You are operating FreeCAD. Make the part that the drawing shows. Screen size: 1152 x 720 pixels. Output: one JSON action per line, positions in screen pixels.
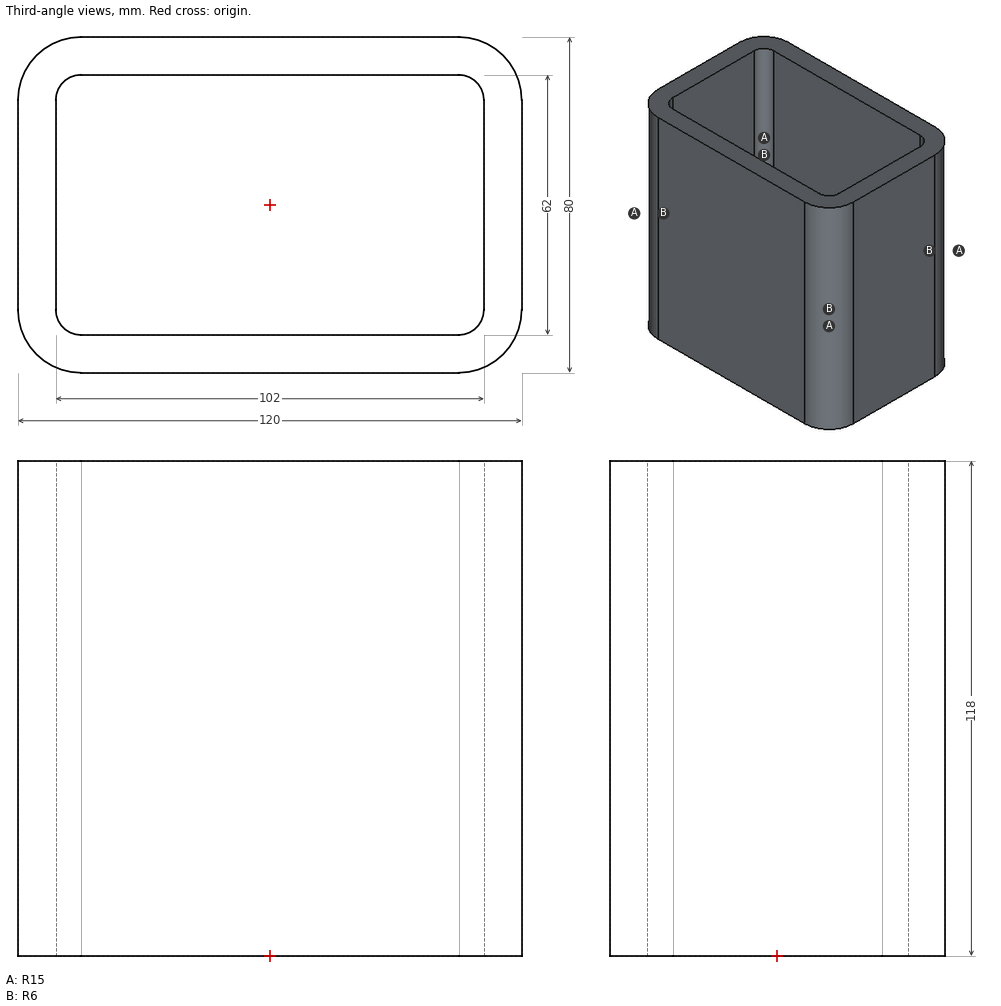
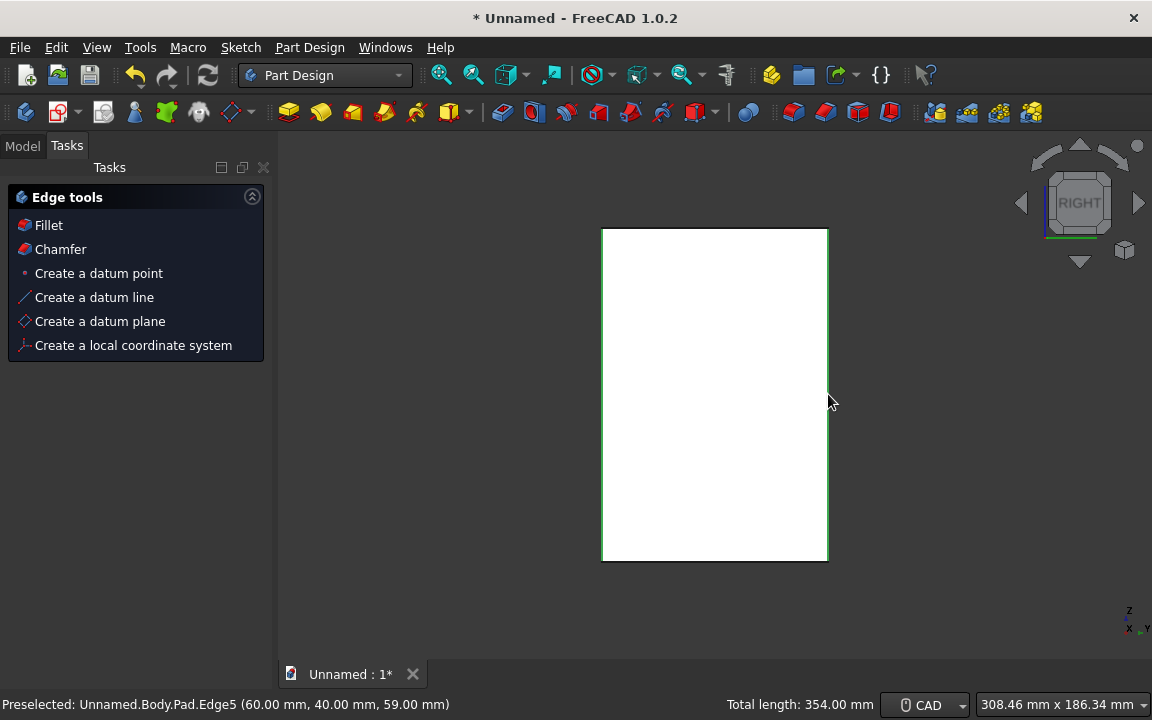
{"action": "key", "text": "5"}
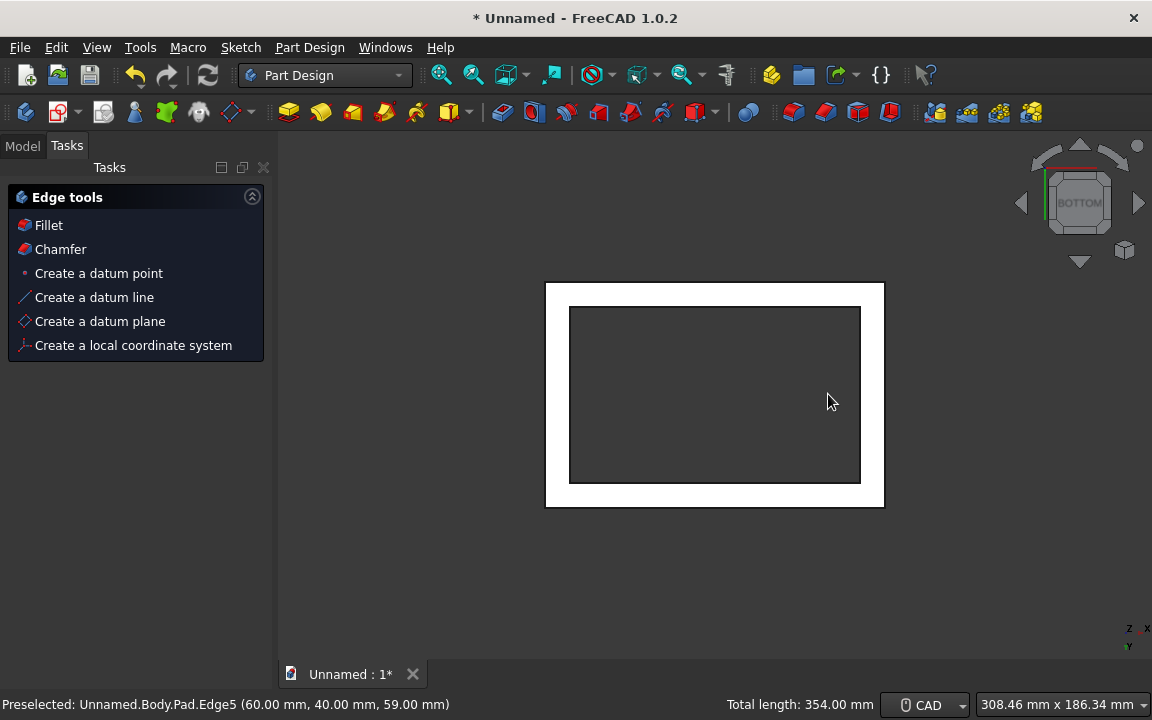
{"action": "left_click", "coordinate": [442, 76]}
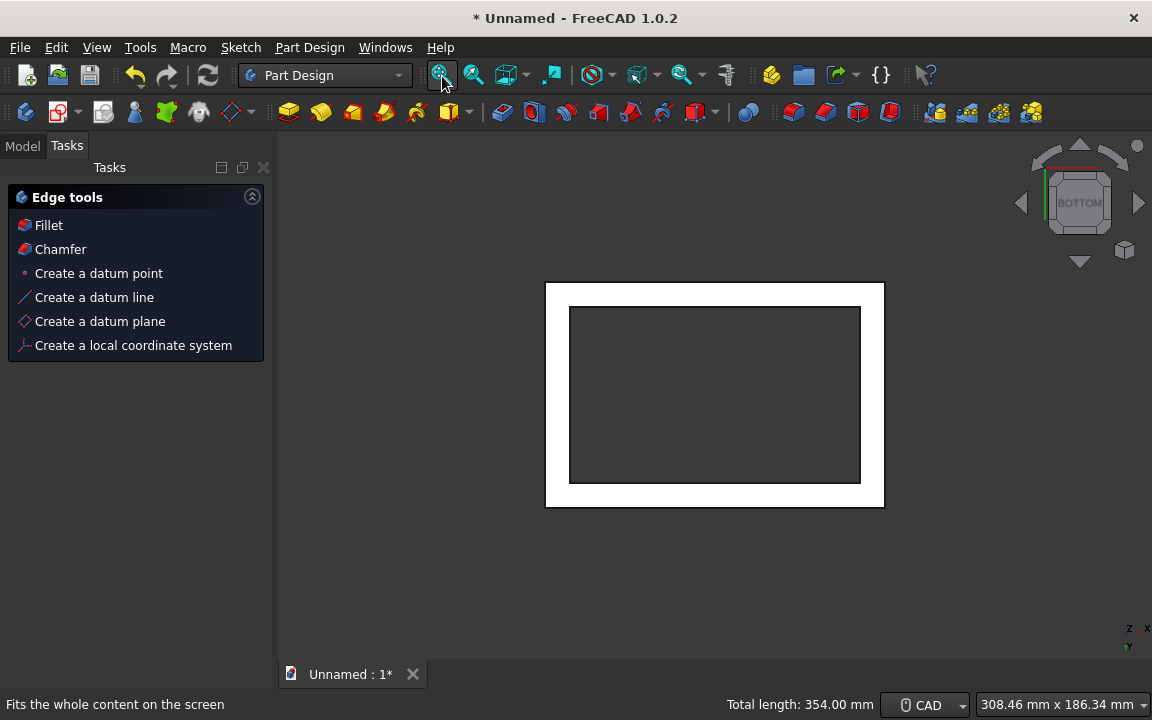
{"action": "key", "text": "4"}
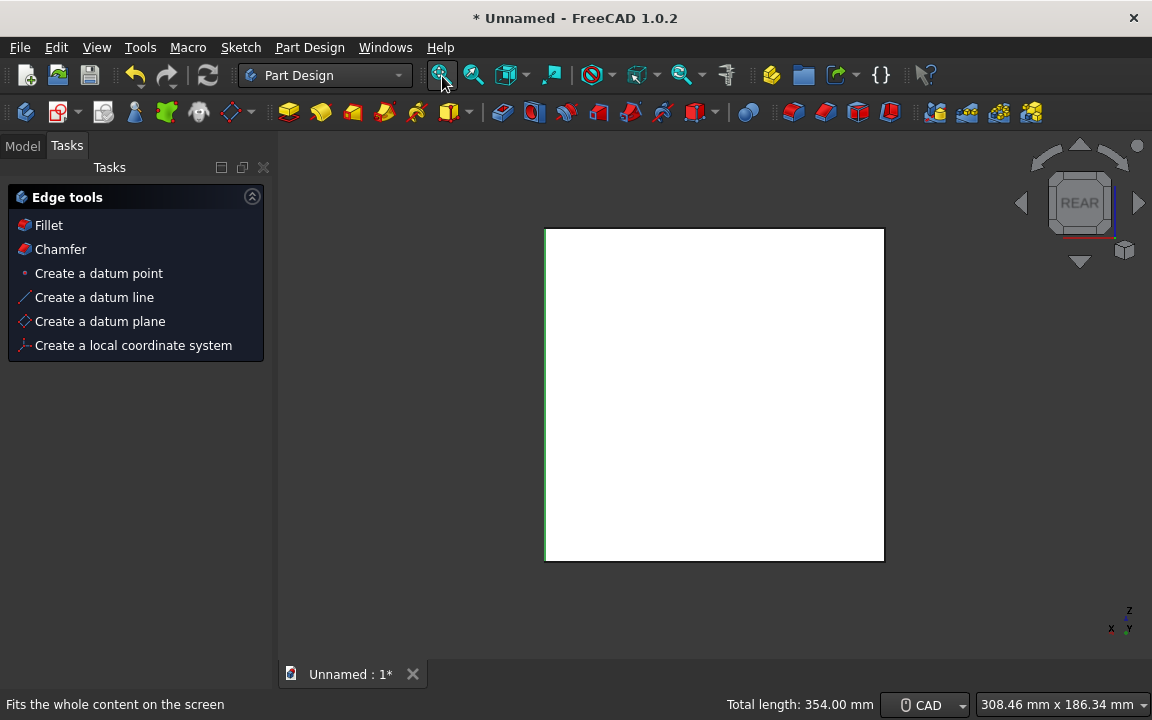
{"action": "left_click", "coordinate": [885, 394], "text": "ctrl"}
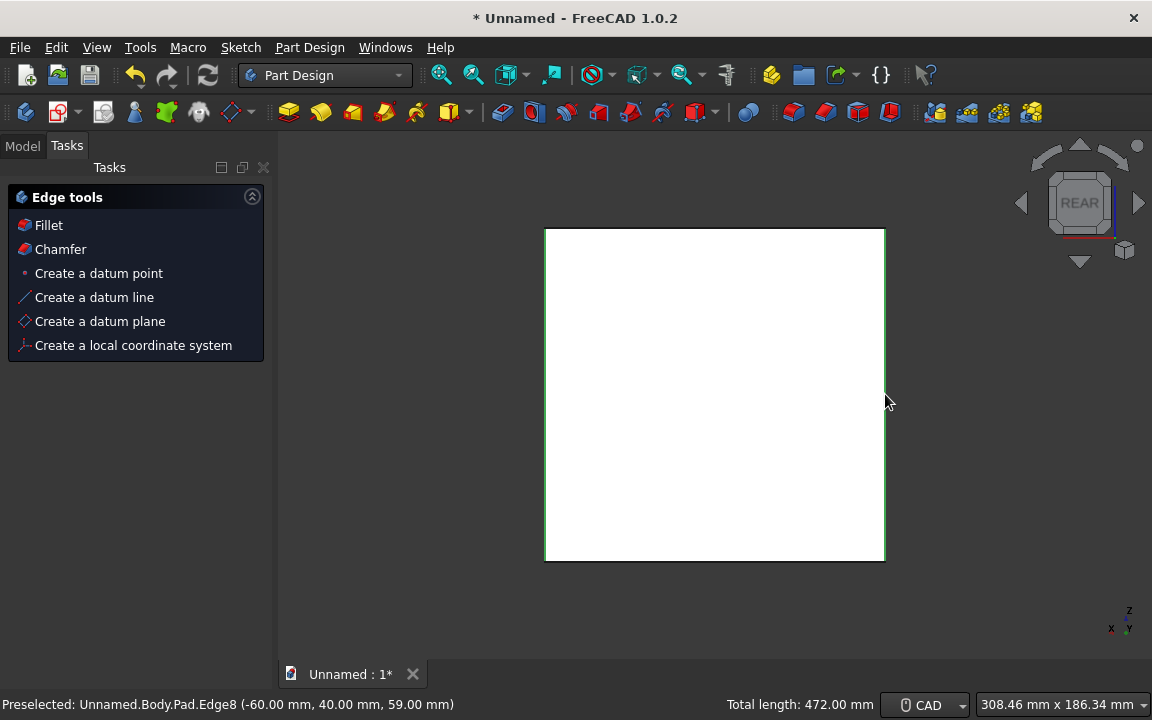
{"action": "left_click", "coordinate": [794, 112]}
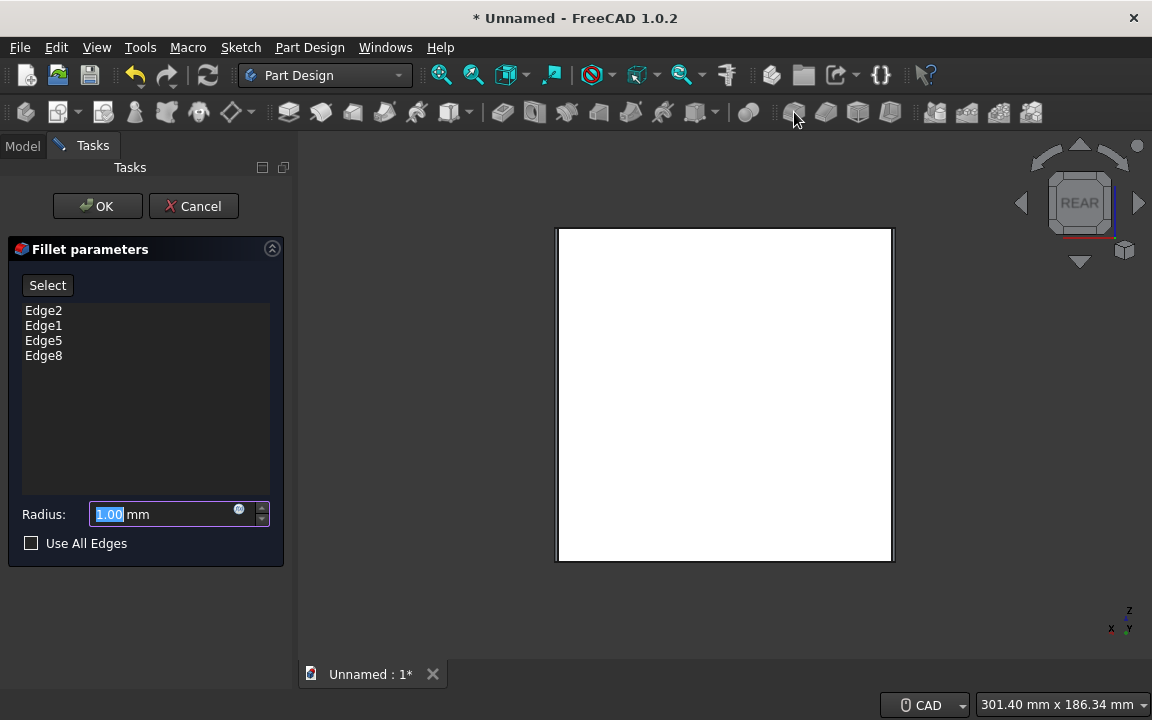
{"action": "type", "text": "15"}
{"action": "key", "text": "Tab"}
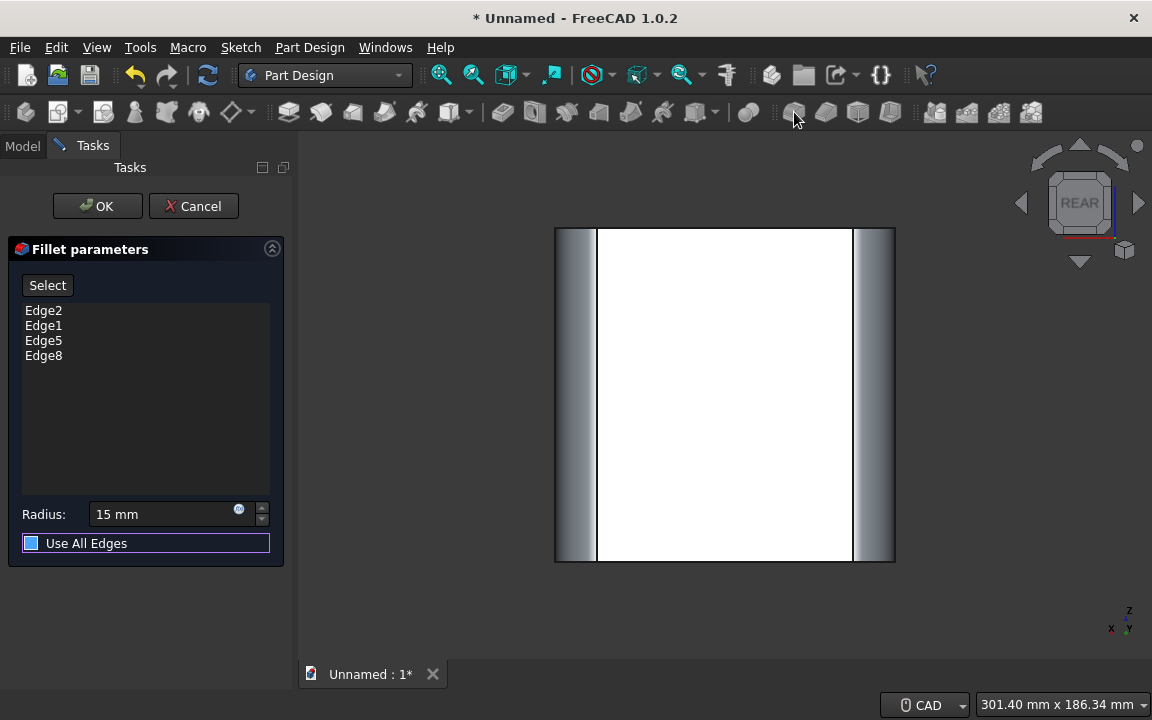
{"action": "left_click", "coordinate": [98, 206]}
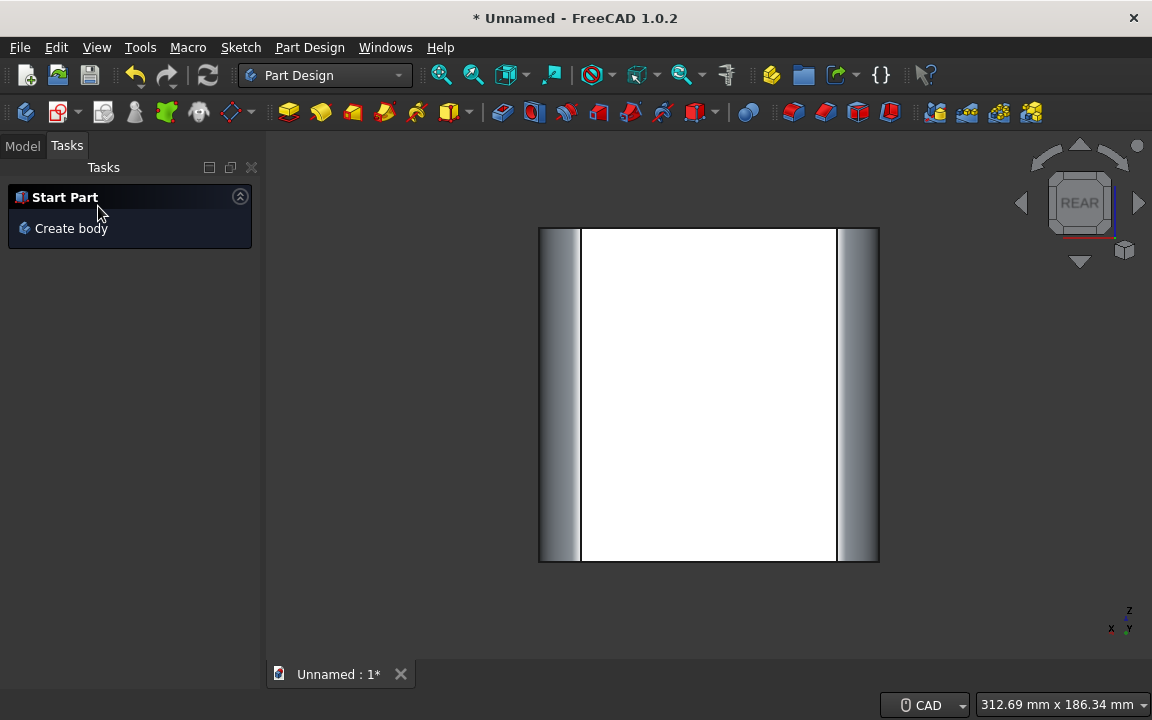
{"action": "key", "text": "0"}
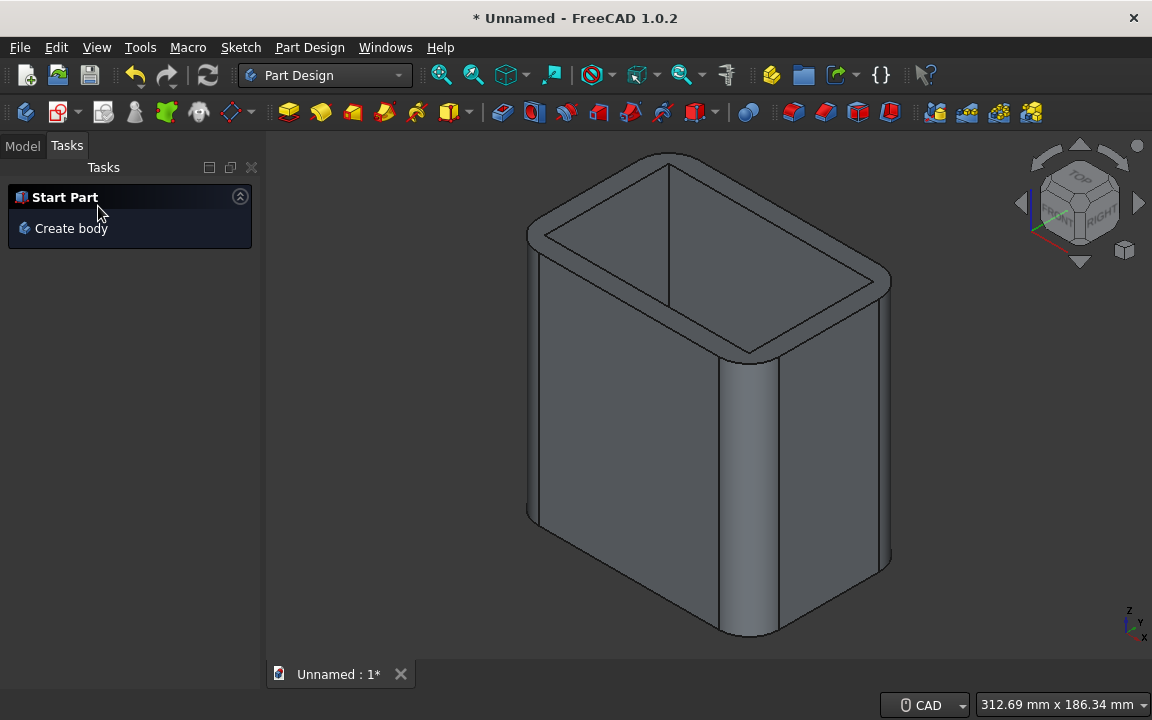
{"action": "key", "text": "2"}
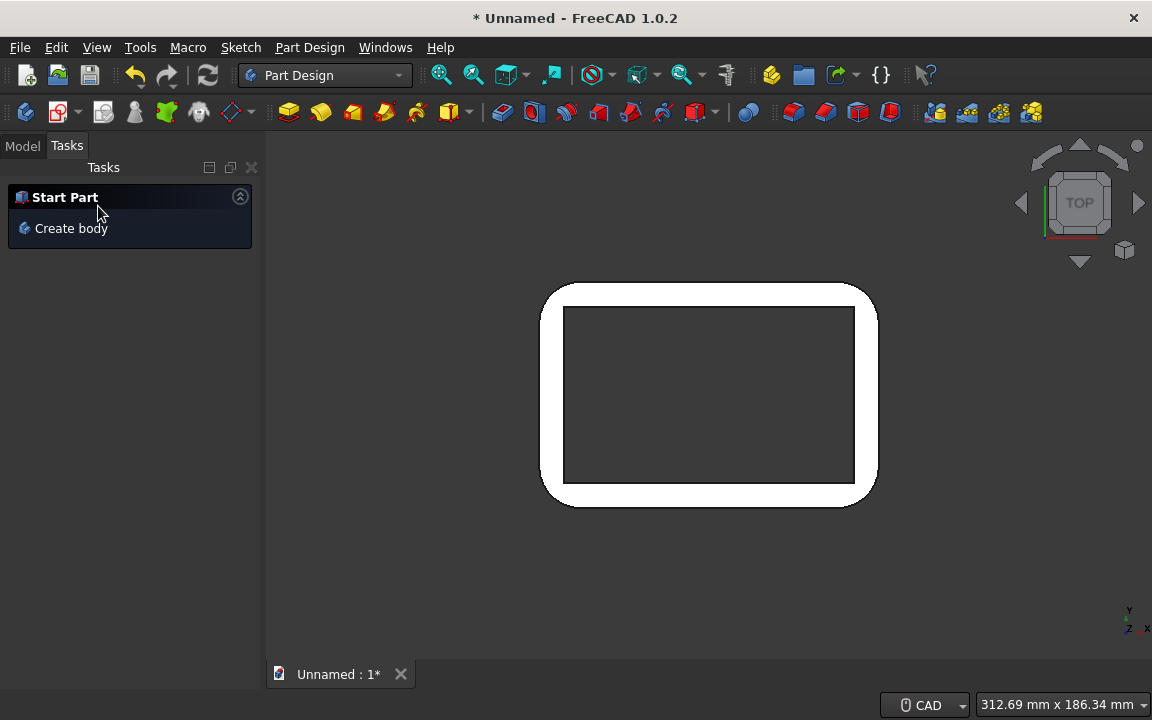
{"action": "left_click", "coordinate": [442, 76]}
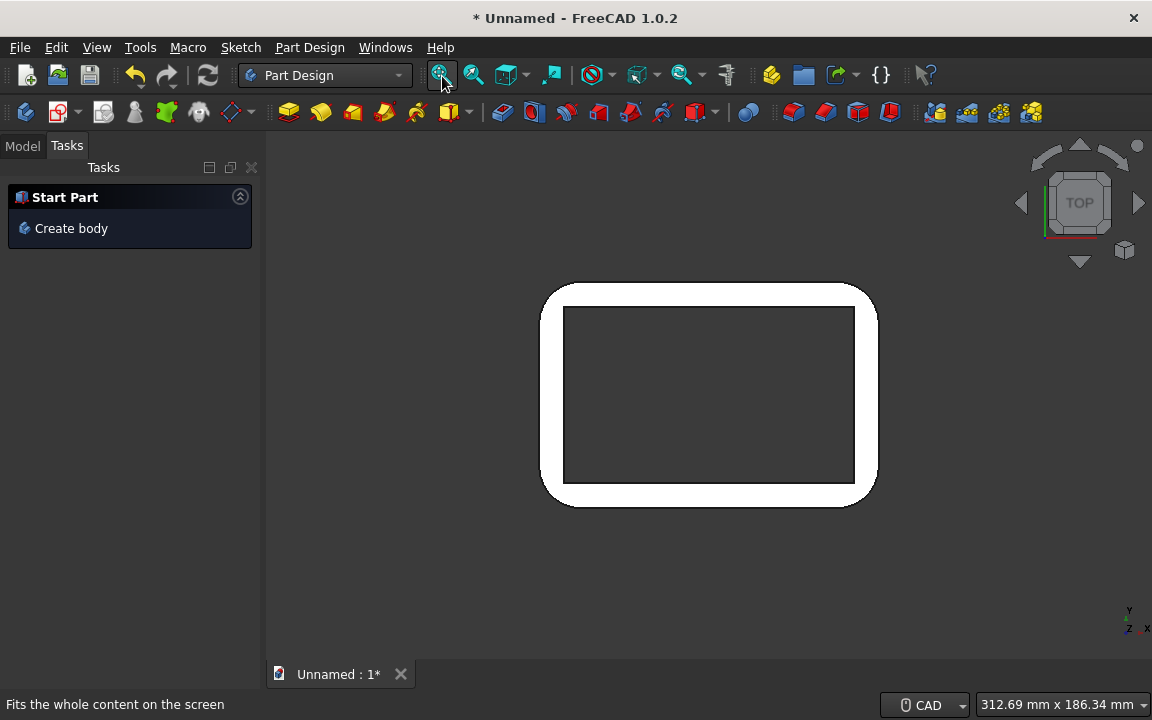
{"action": "key", "text": "1"}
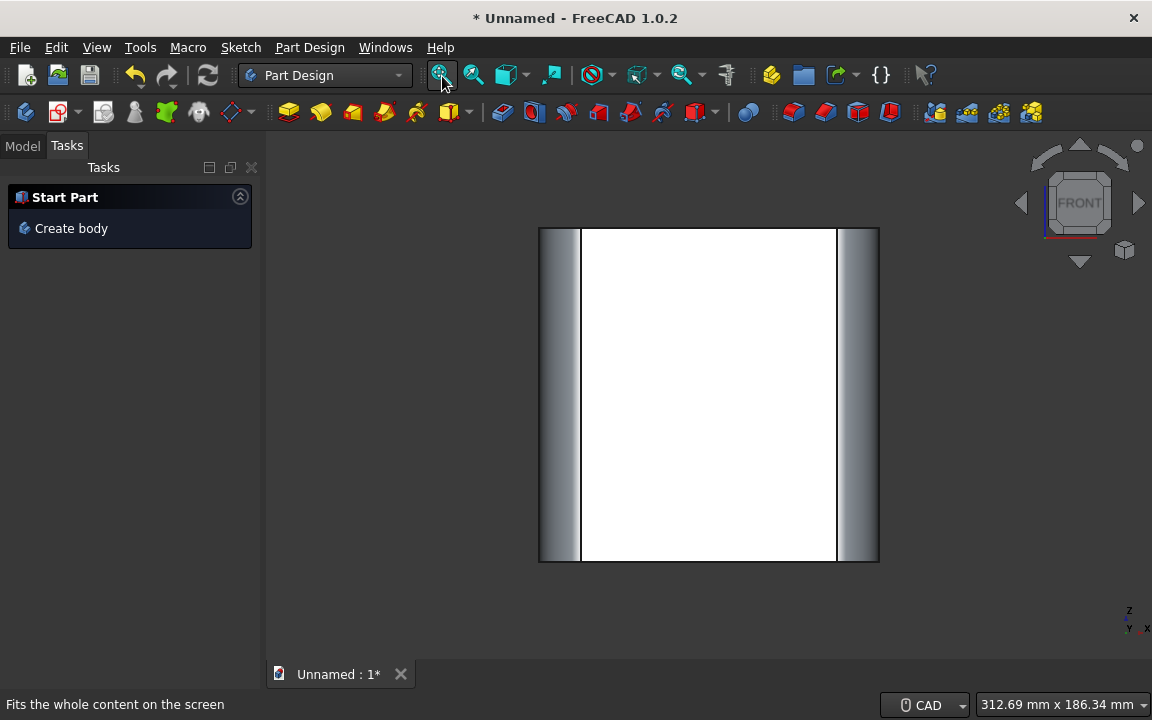
{"action": "key", "text": "3"}